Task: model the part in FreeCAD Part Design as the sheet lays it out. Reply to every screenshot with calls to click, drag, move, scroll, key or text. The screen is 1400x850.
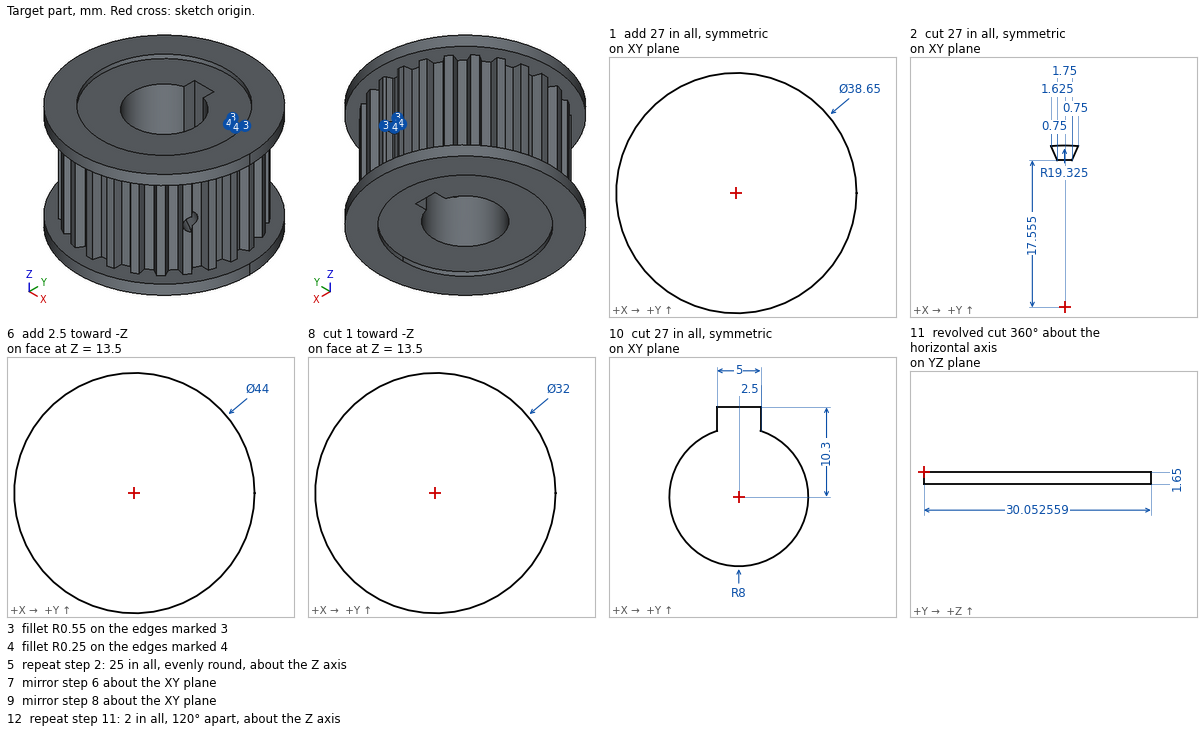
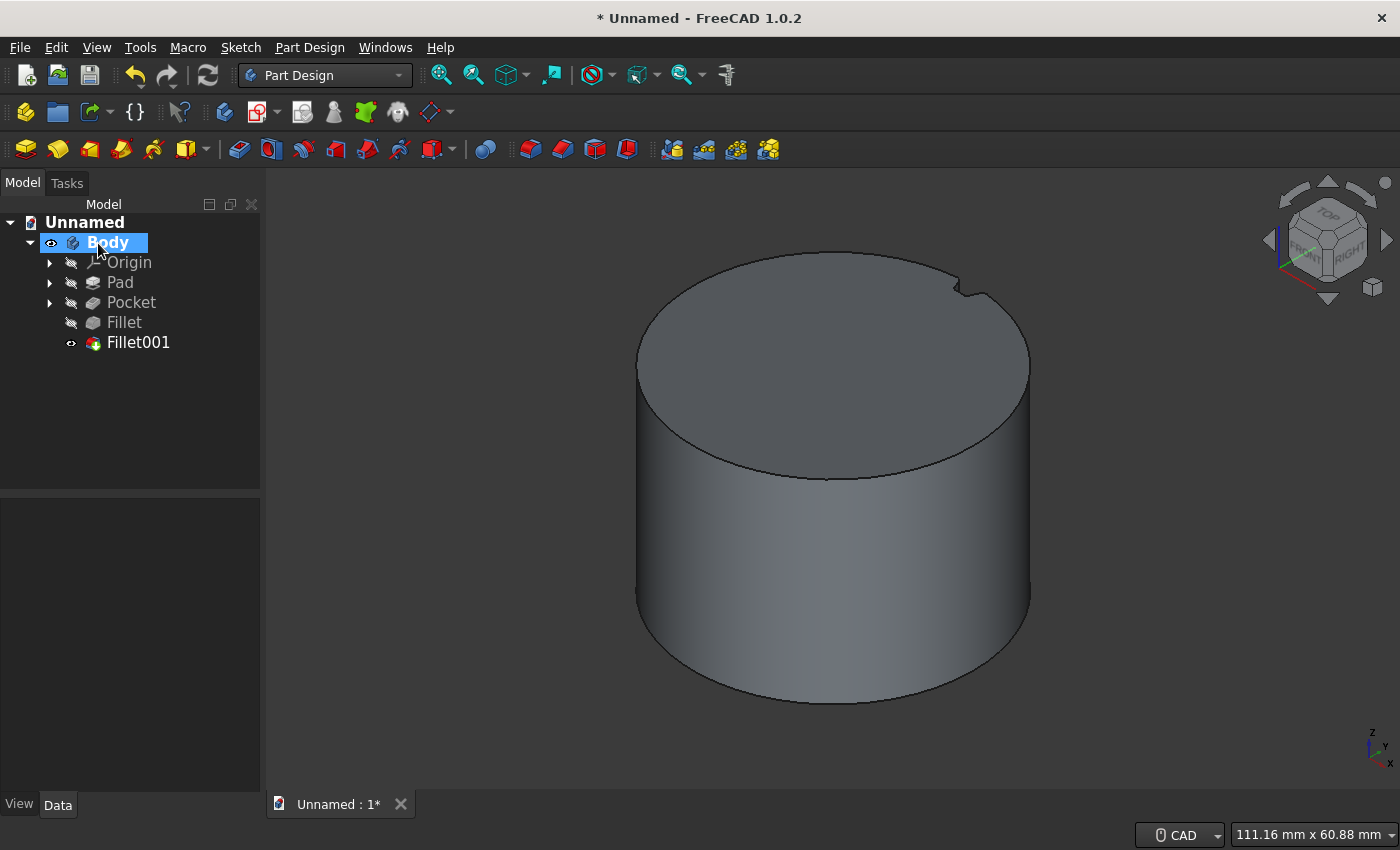
click(116, 303)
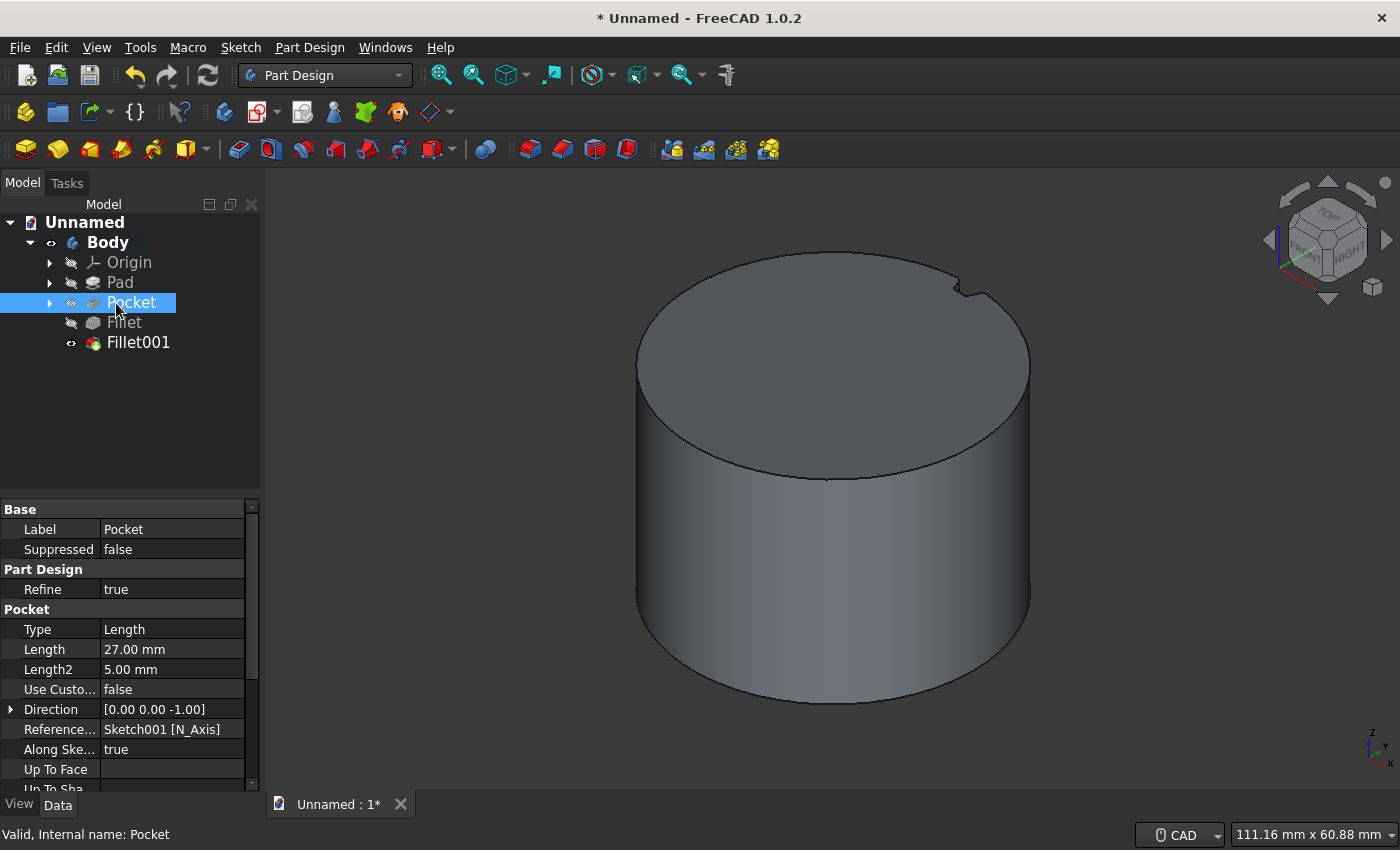
click(736, 150)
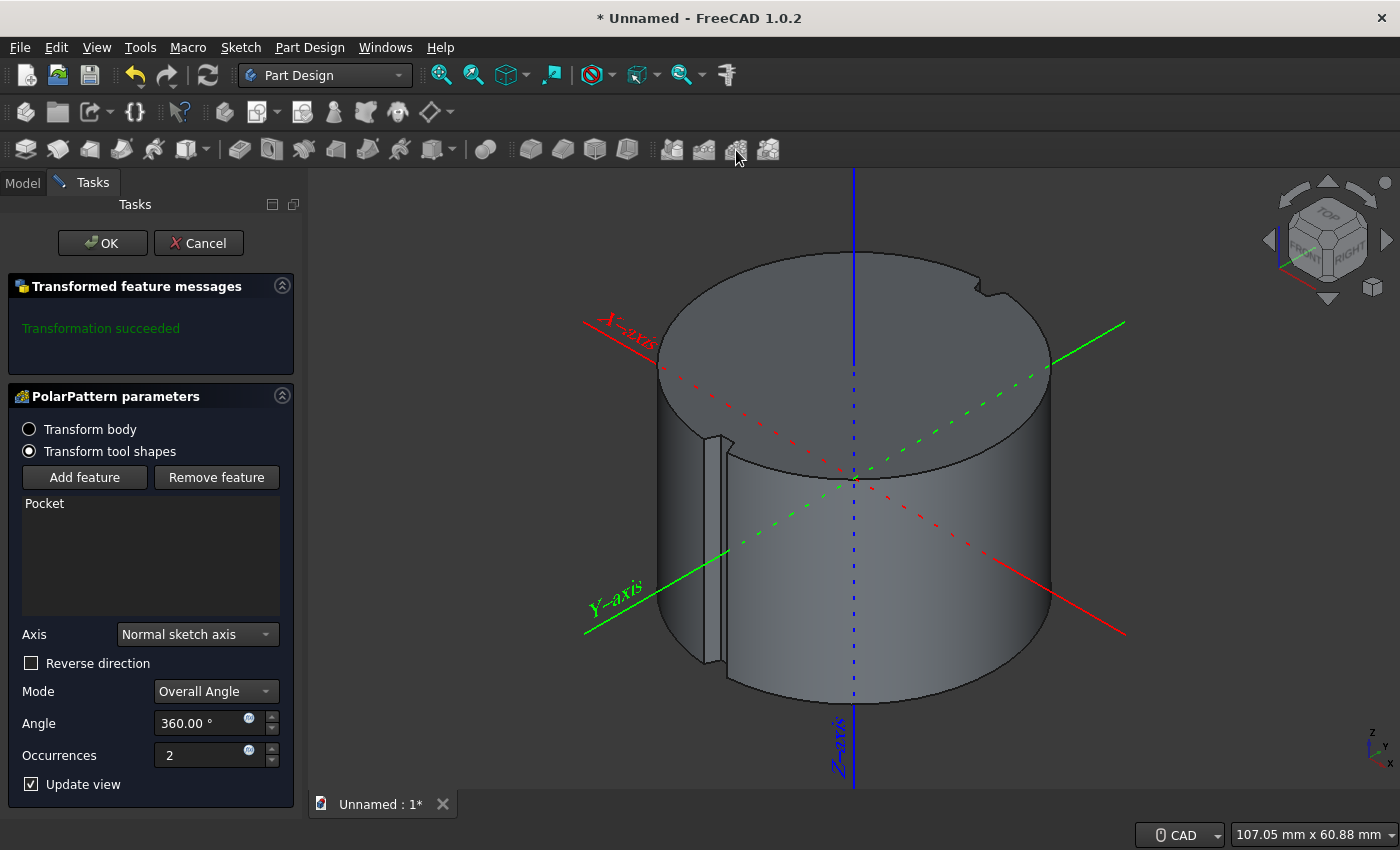
click(198, 634)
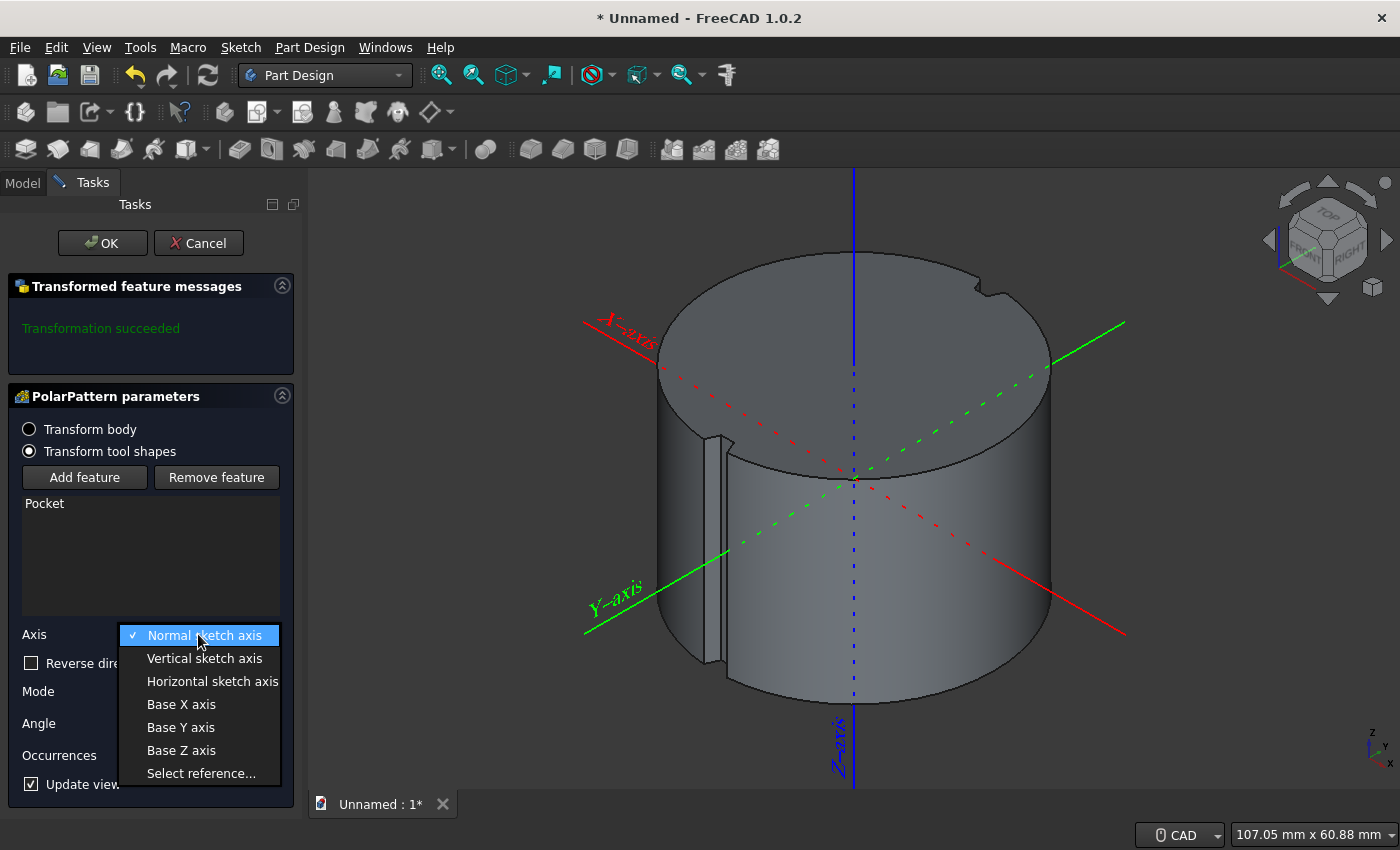
click(198, 750)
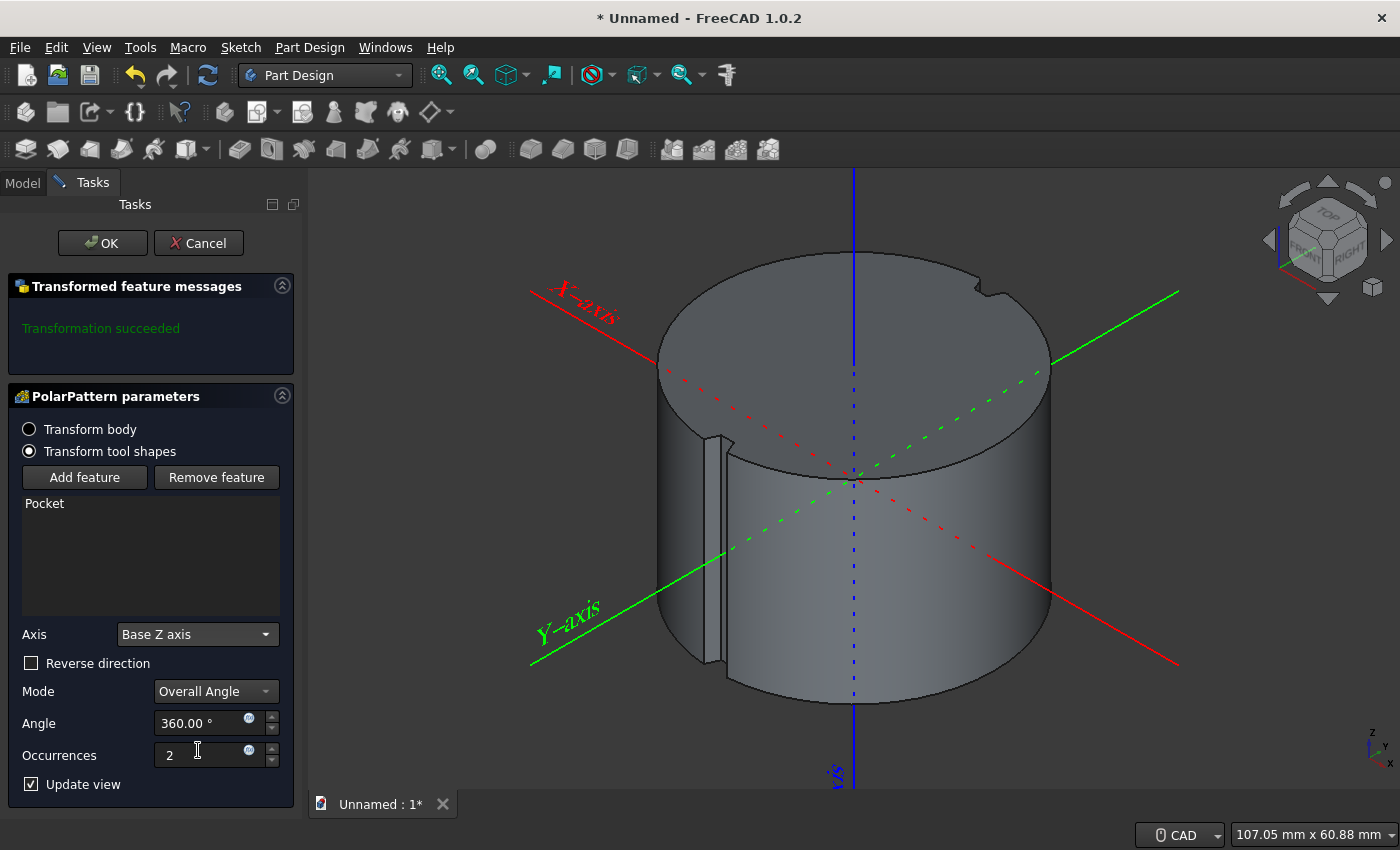
triple_click(209, 755)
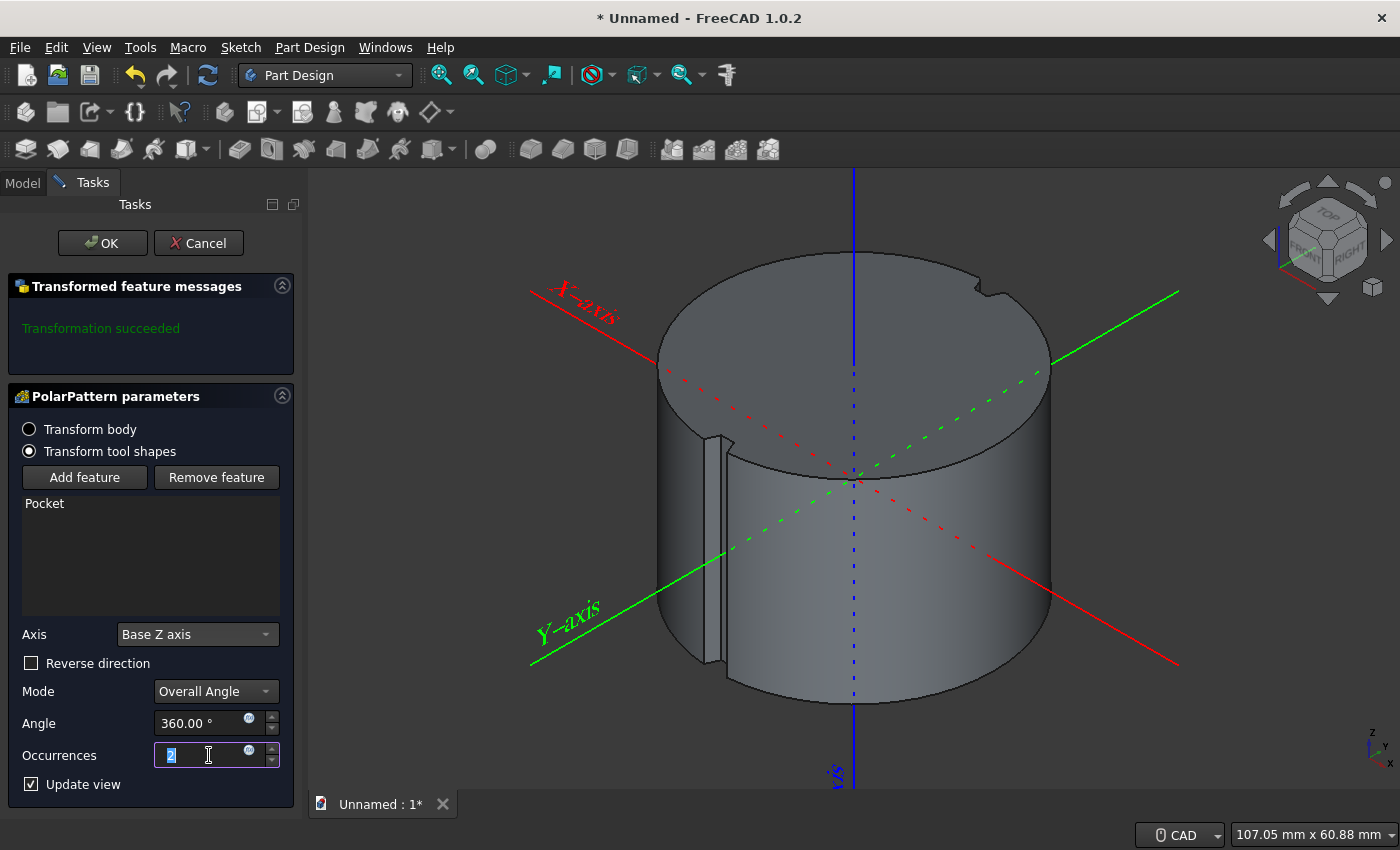
text(25)
key(Tab)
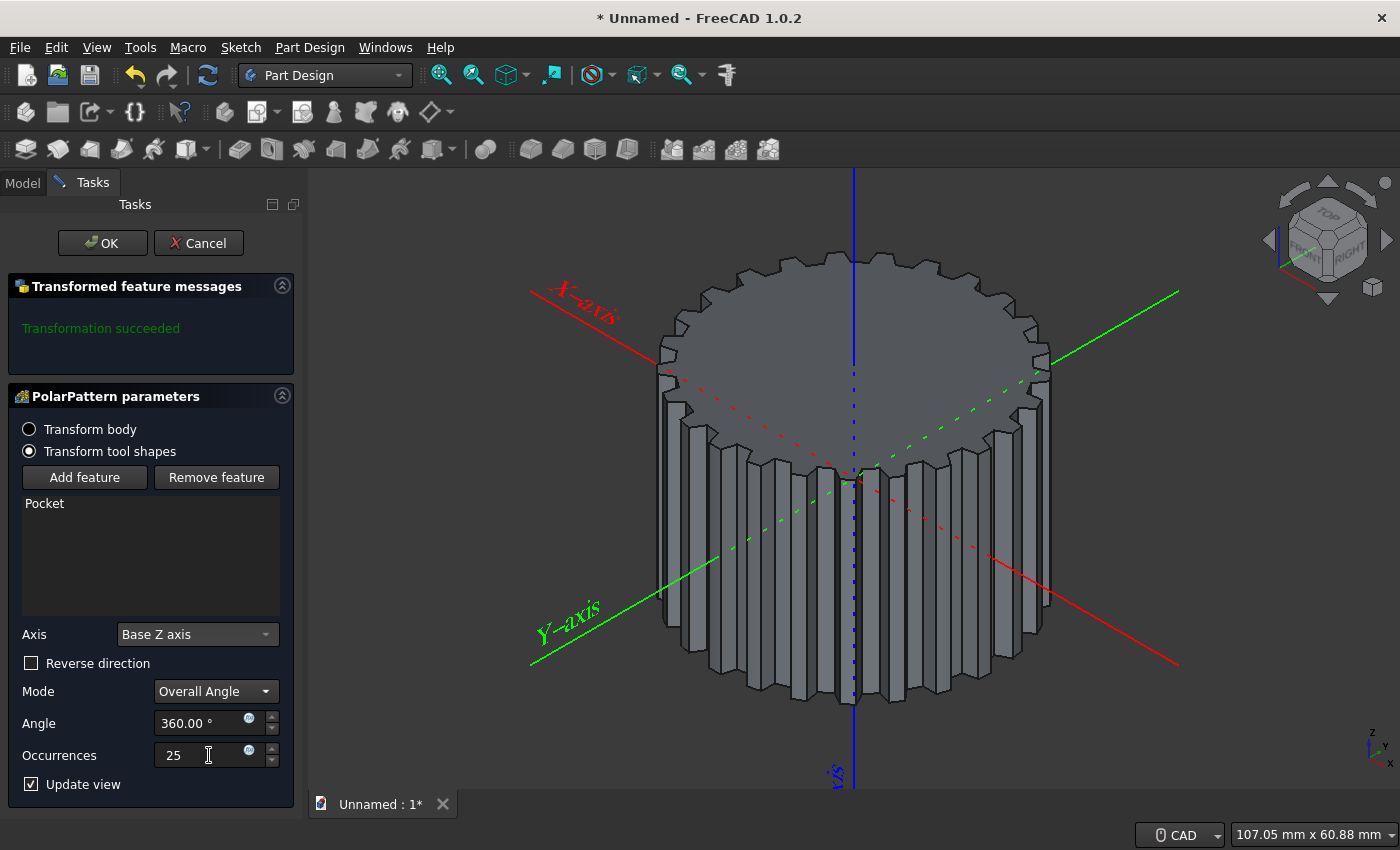
click(103, 243)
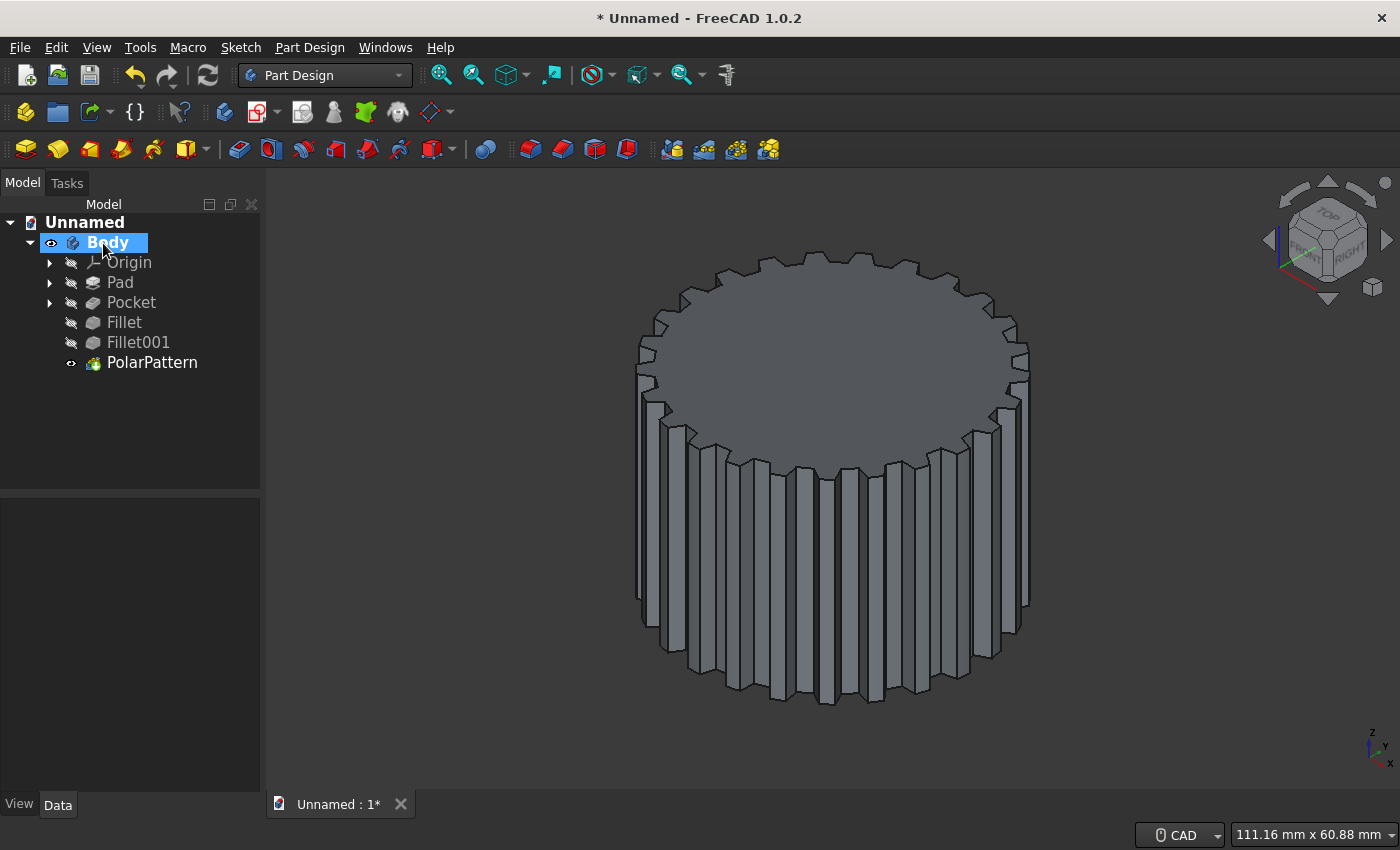
click(833, 365)